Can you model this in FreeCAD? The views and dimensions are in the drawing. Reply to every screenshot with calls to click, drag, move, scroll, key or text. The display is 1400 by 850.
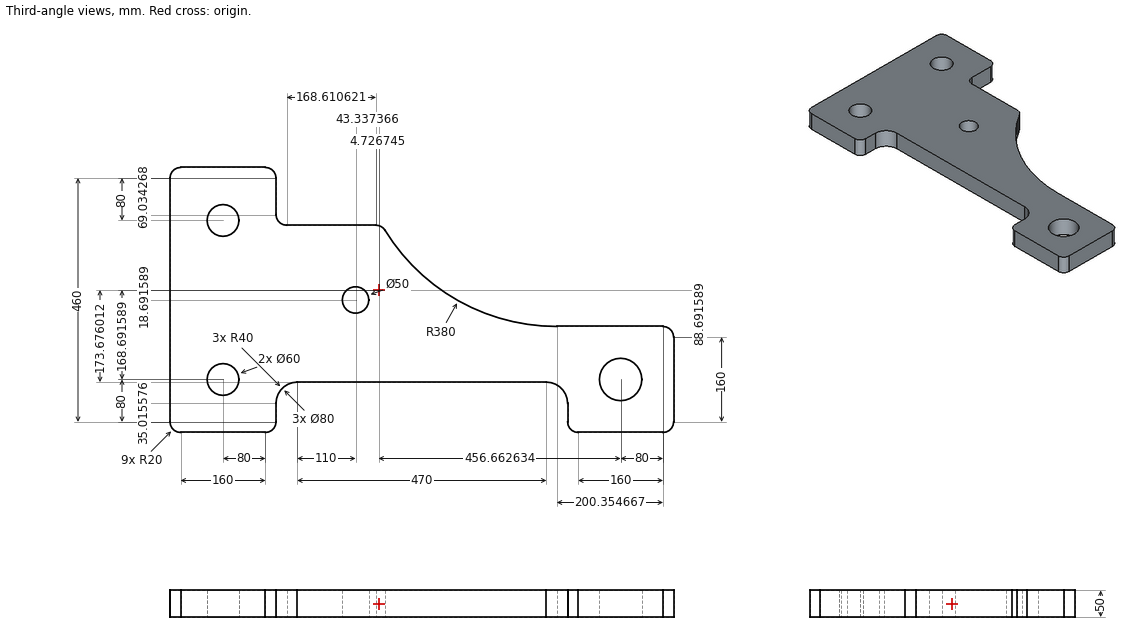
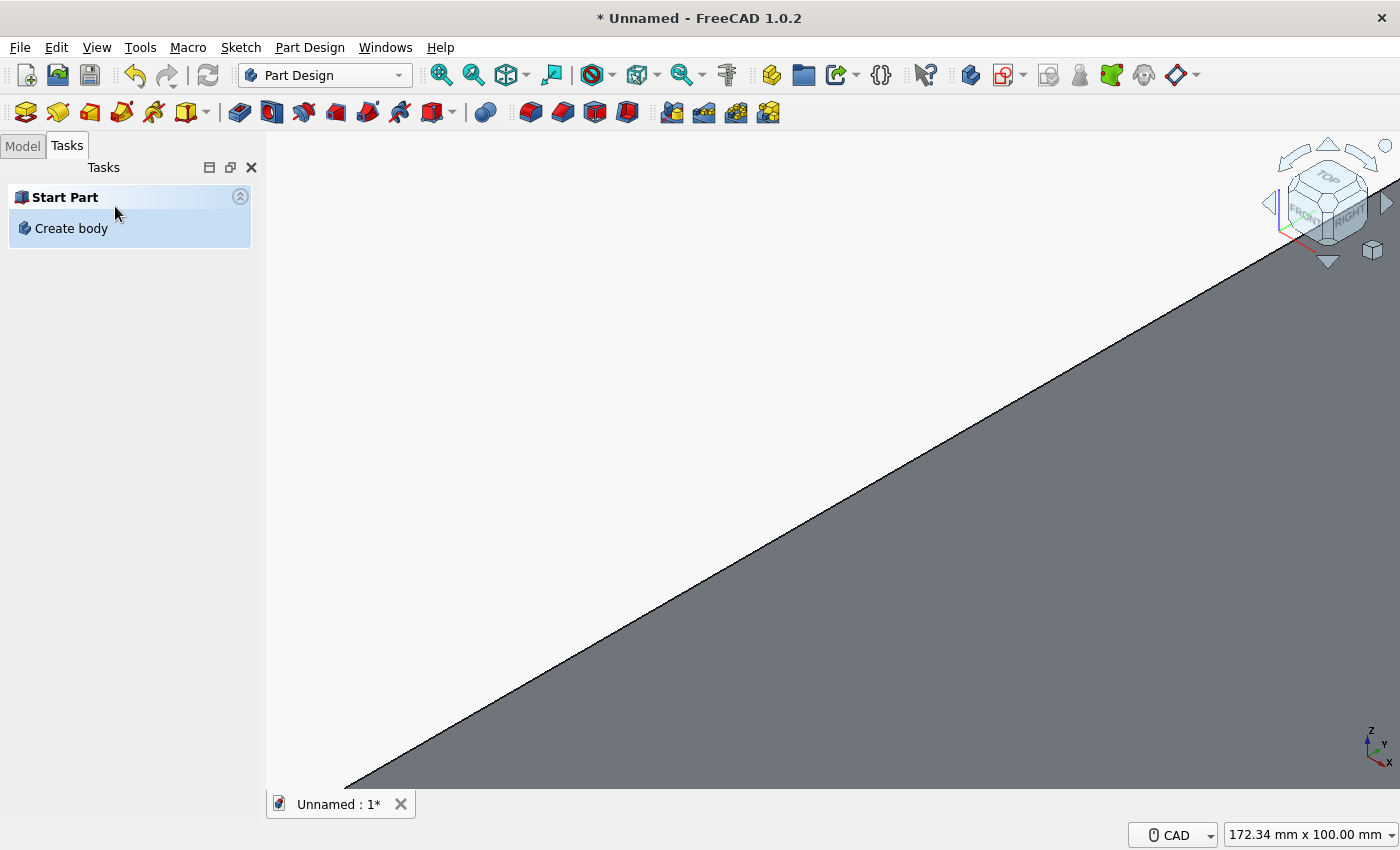
click(442, 76)